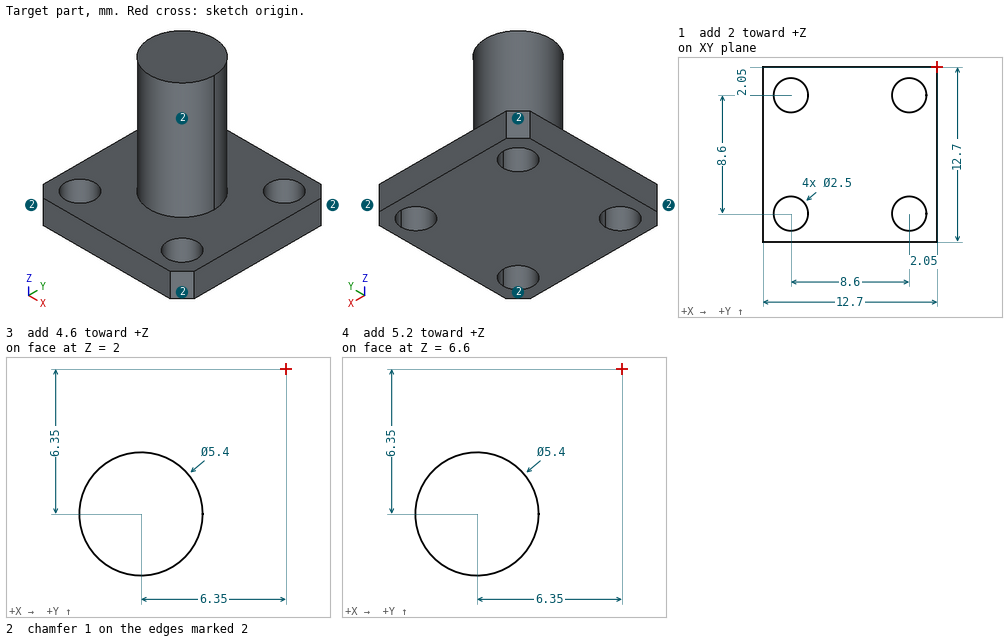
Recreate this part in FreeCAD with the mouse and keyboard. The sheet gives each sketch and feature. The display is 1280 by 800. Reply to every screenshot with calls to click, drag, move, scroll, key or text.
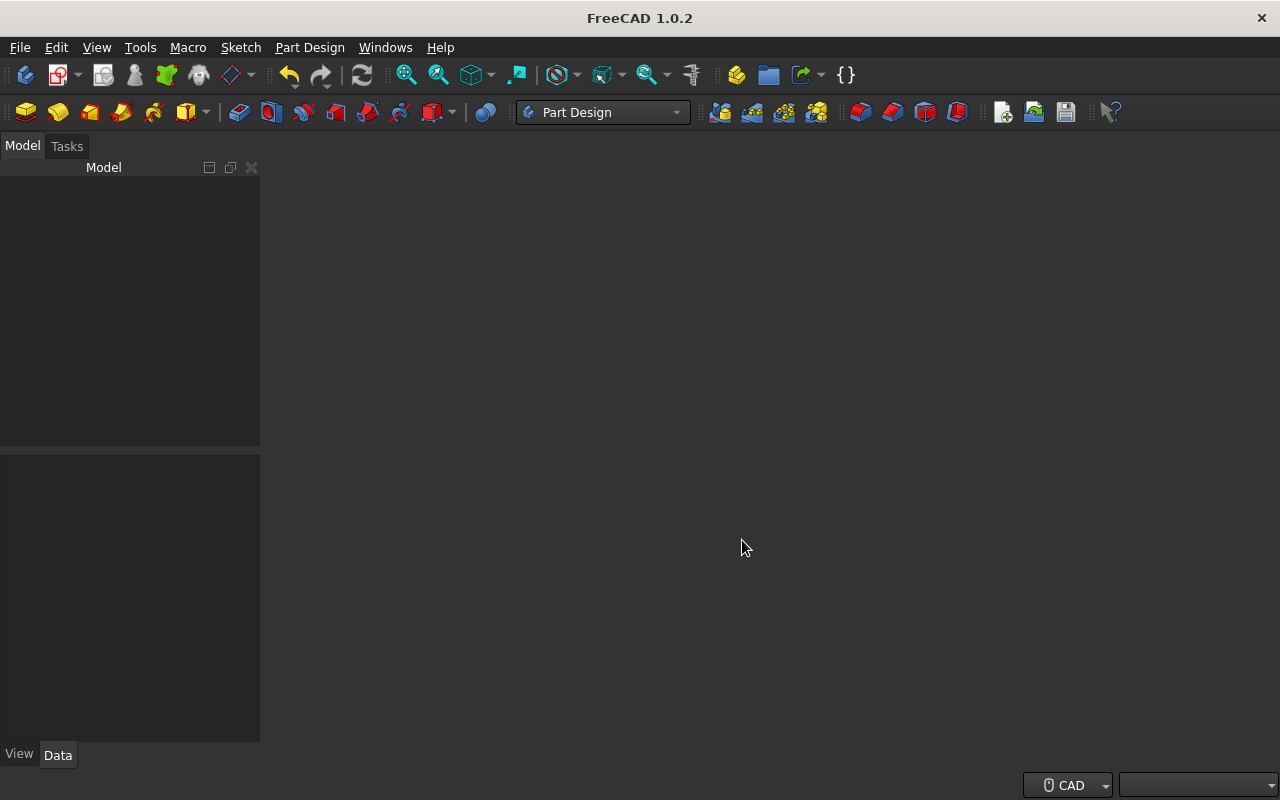
click(1002, 112)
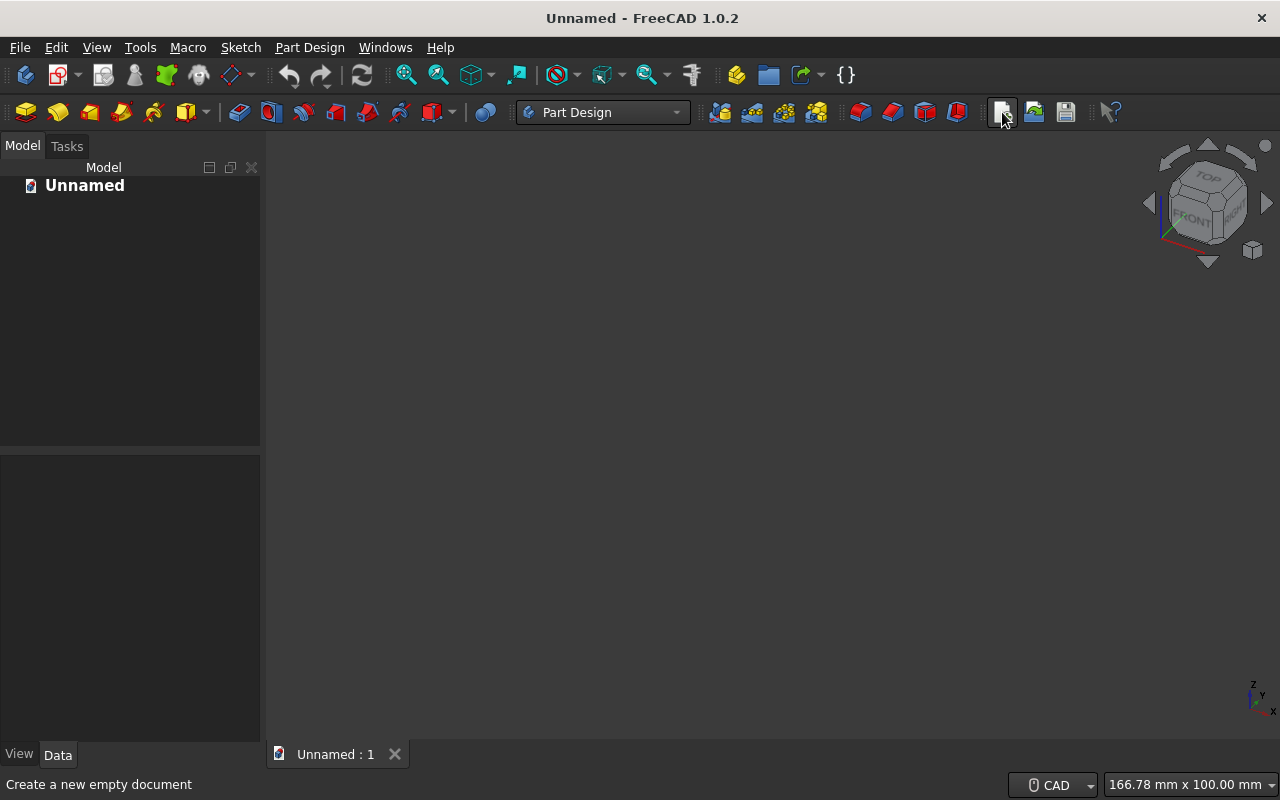
click(58, 76)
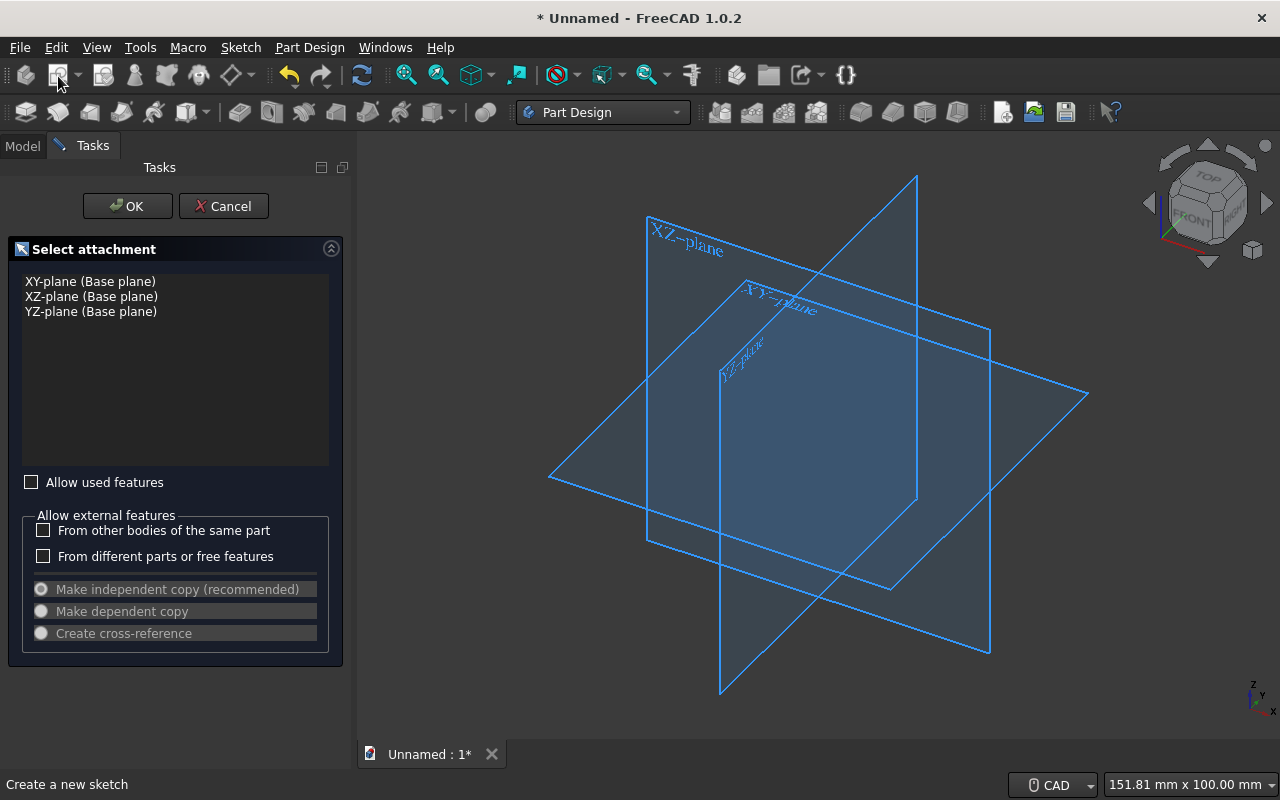
click(82, 282)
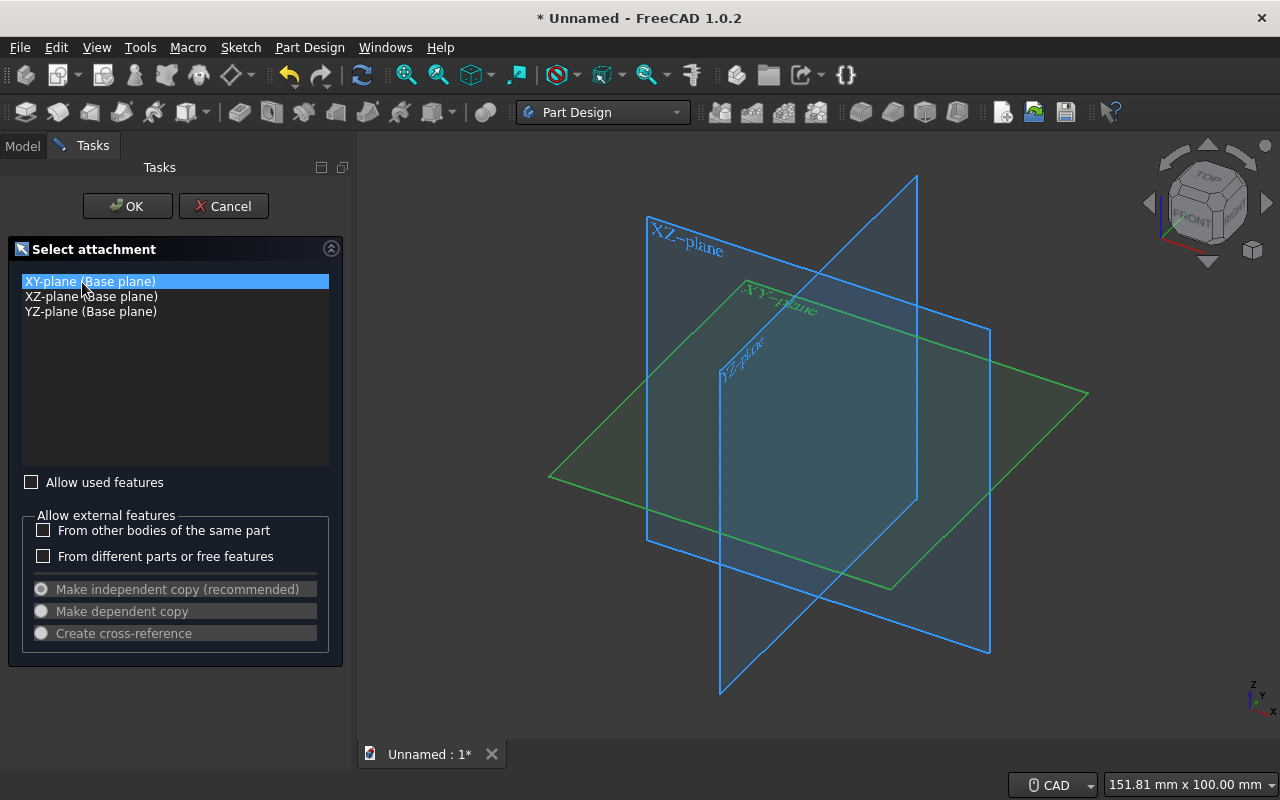
click(128, 206)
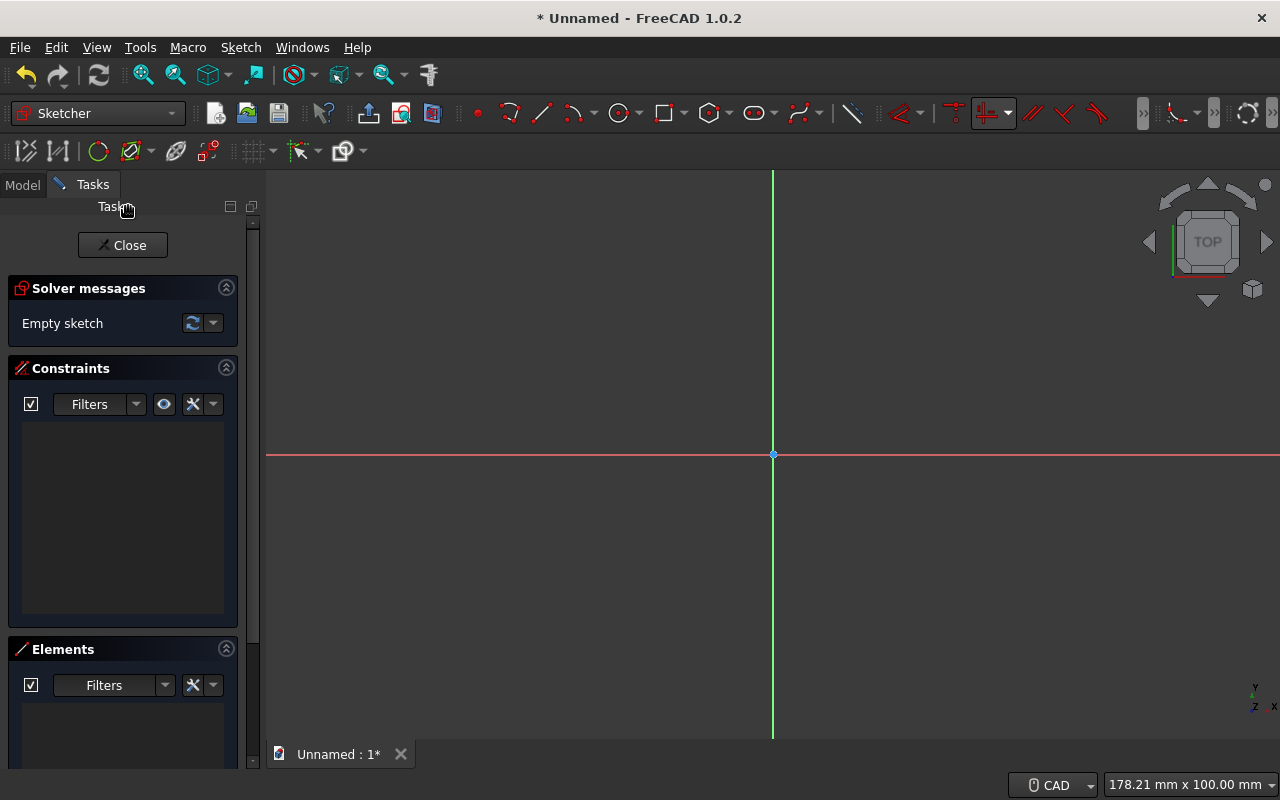
scroll(745, 500, up, 8)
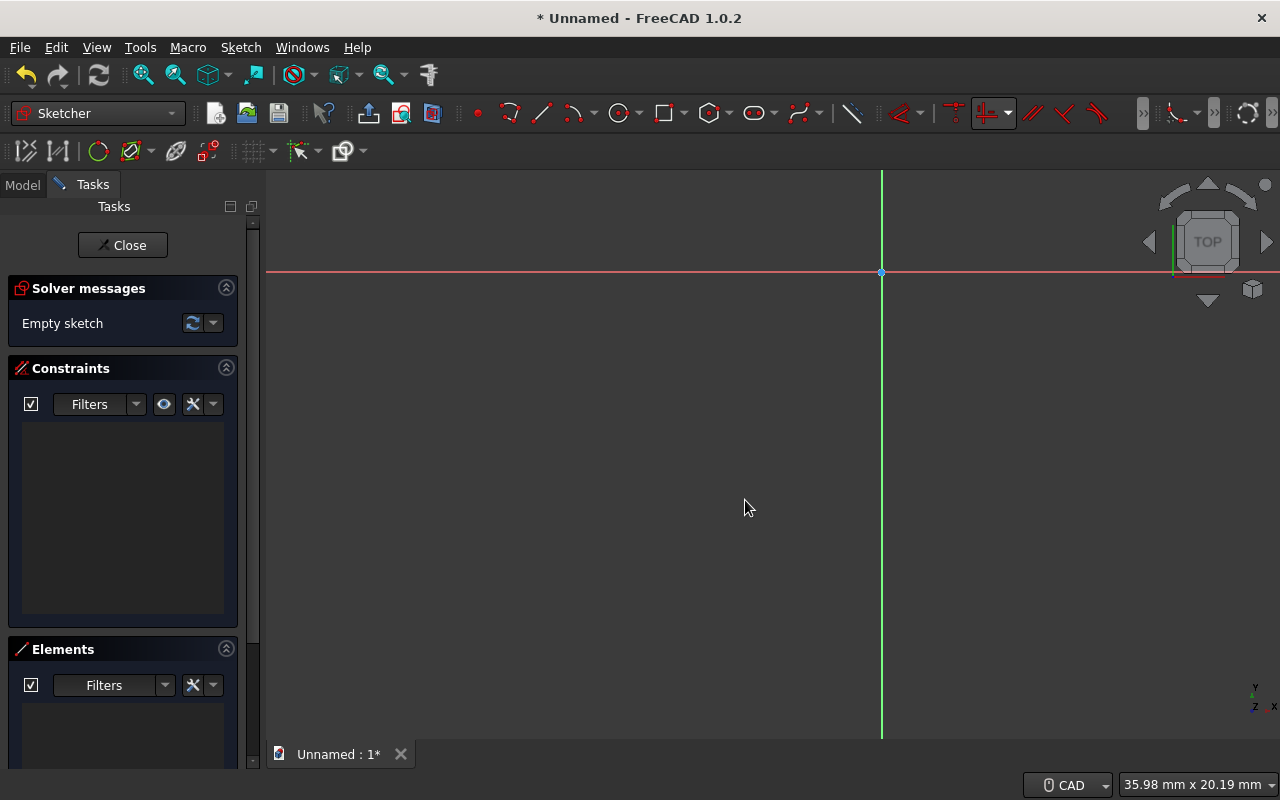
click(664, 114)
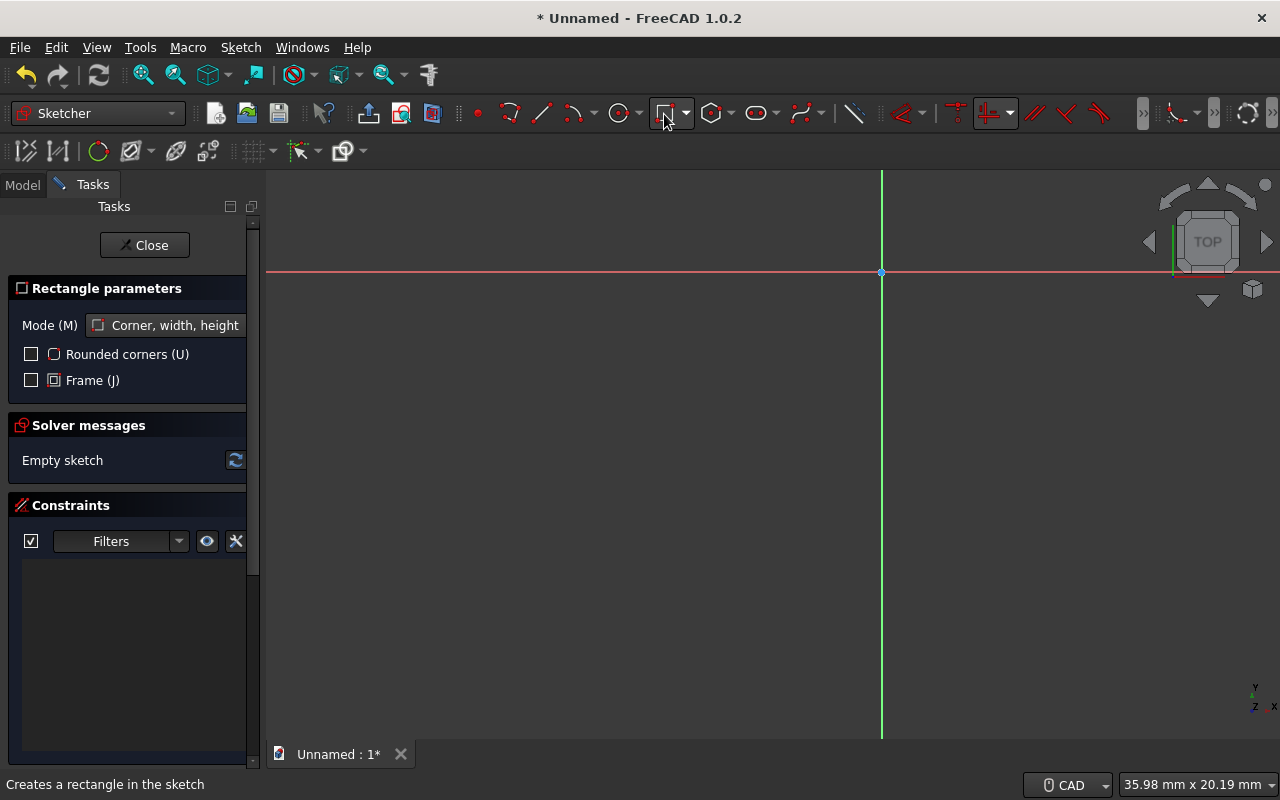
click(882, 272)
move(524, 630)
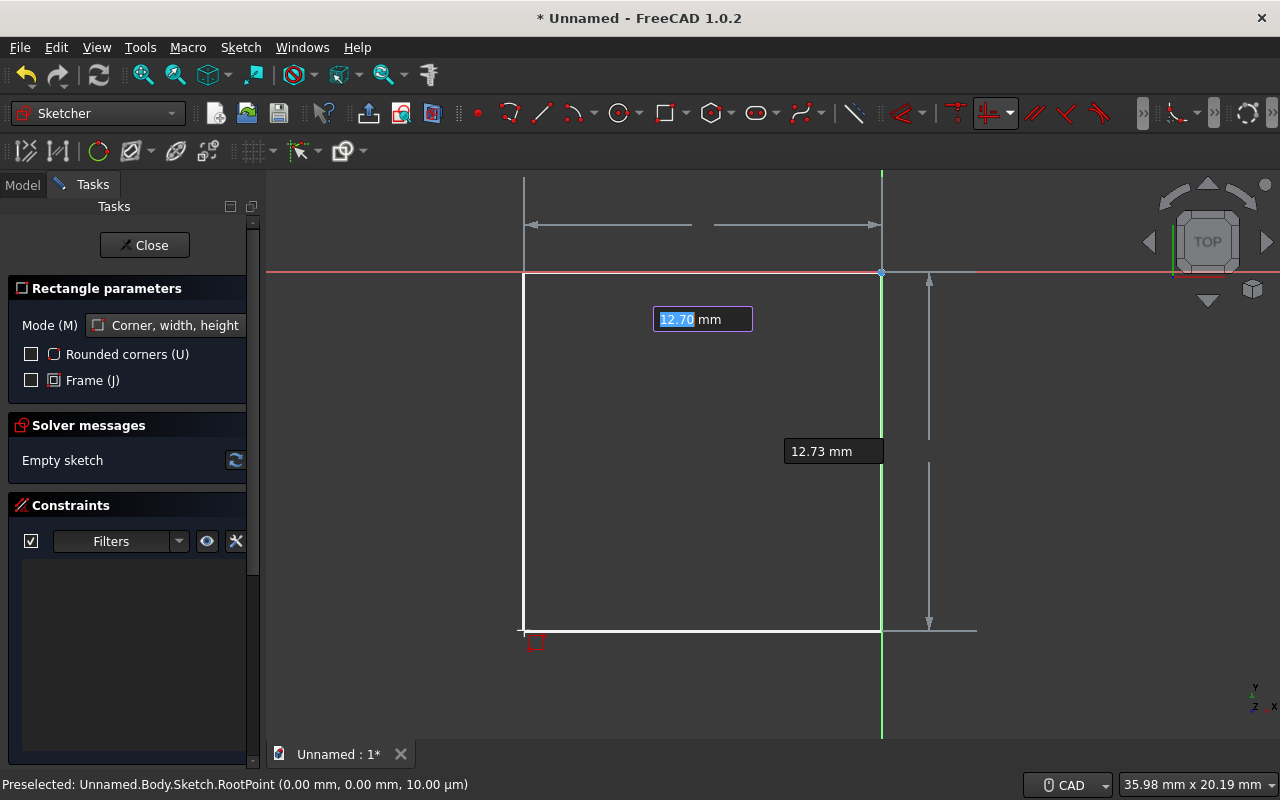
text(12.7)
key(Tab)
text(12.7)
key(Return)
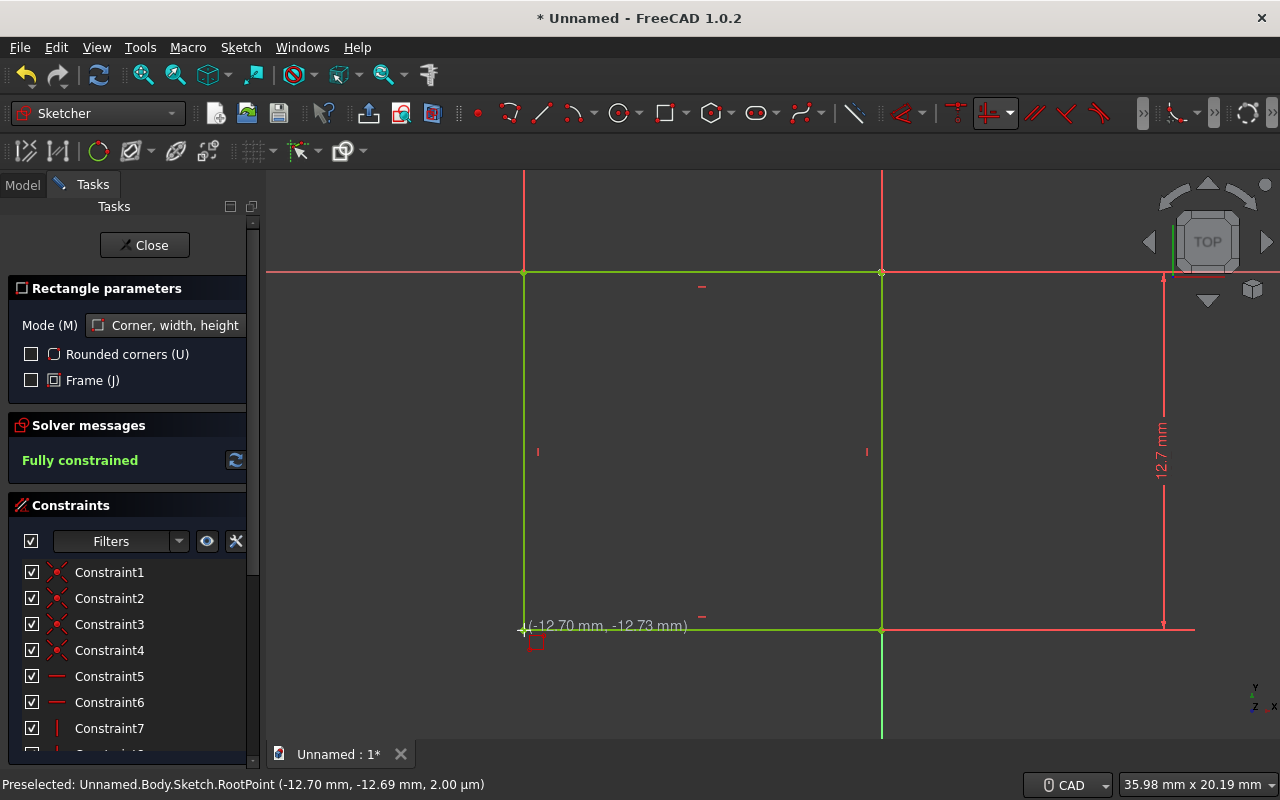
click(620, 114)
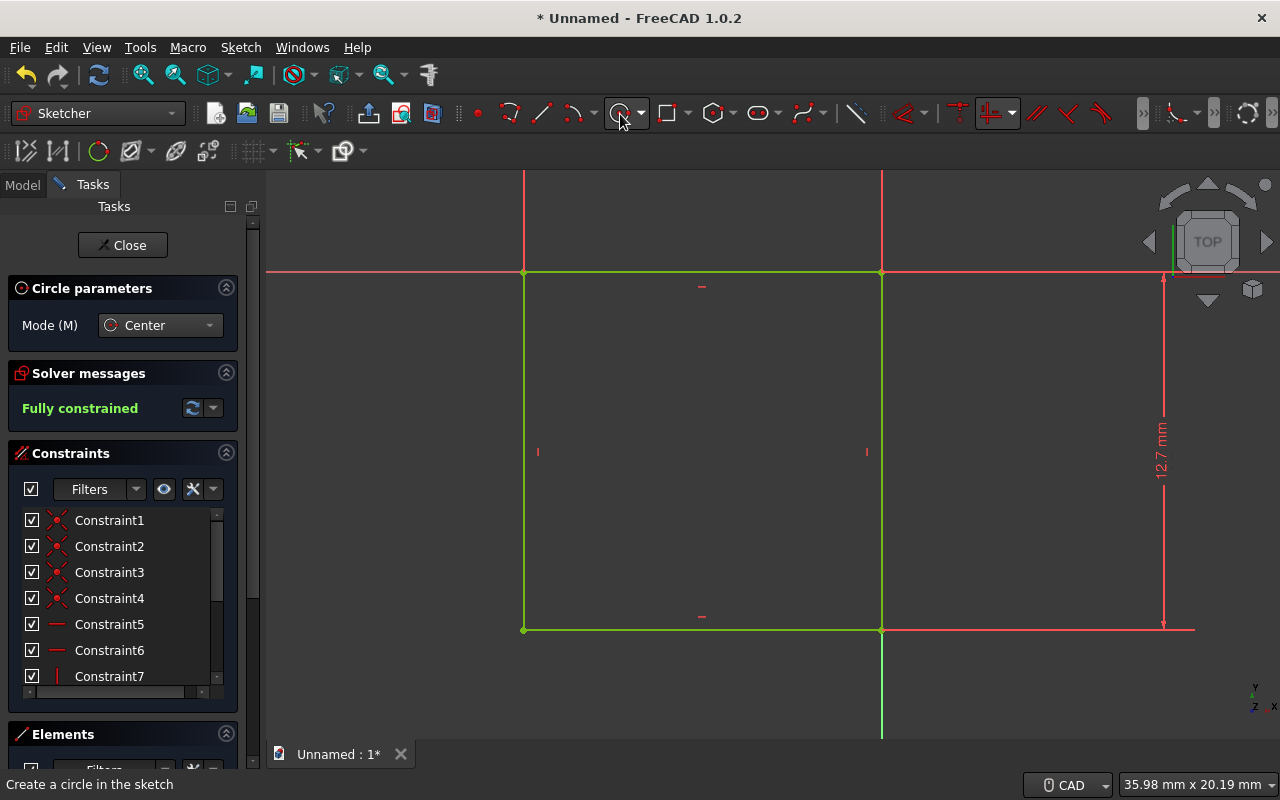
click(582, 572)
move(607, 548)